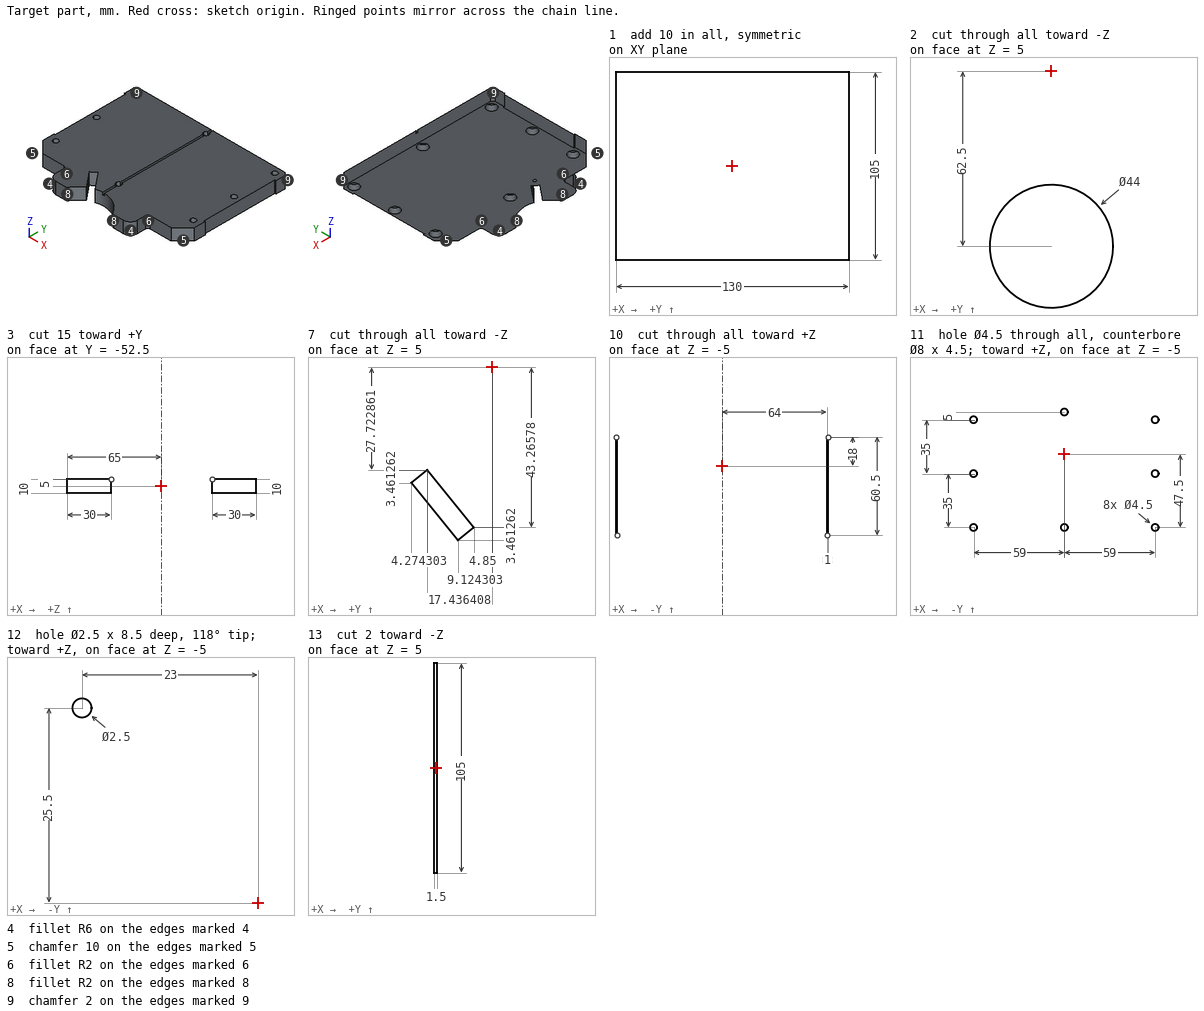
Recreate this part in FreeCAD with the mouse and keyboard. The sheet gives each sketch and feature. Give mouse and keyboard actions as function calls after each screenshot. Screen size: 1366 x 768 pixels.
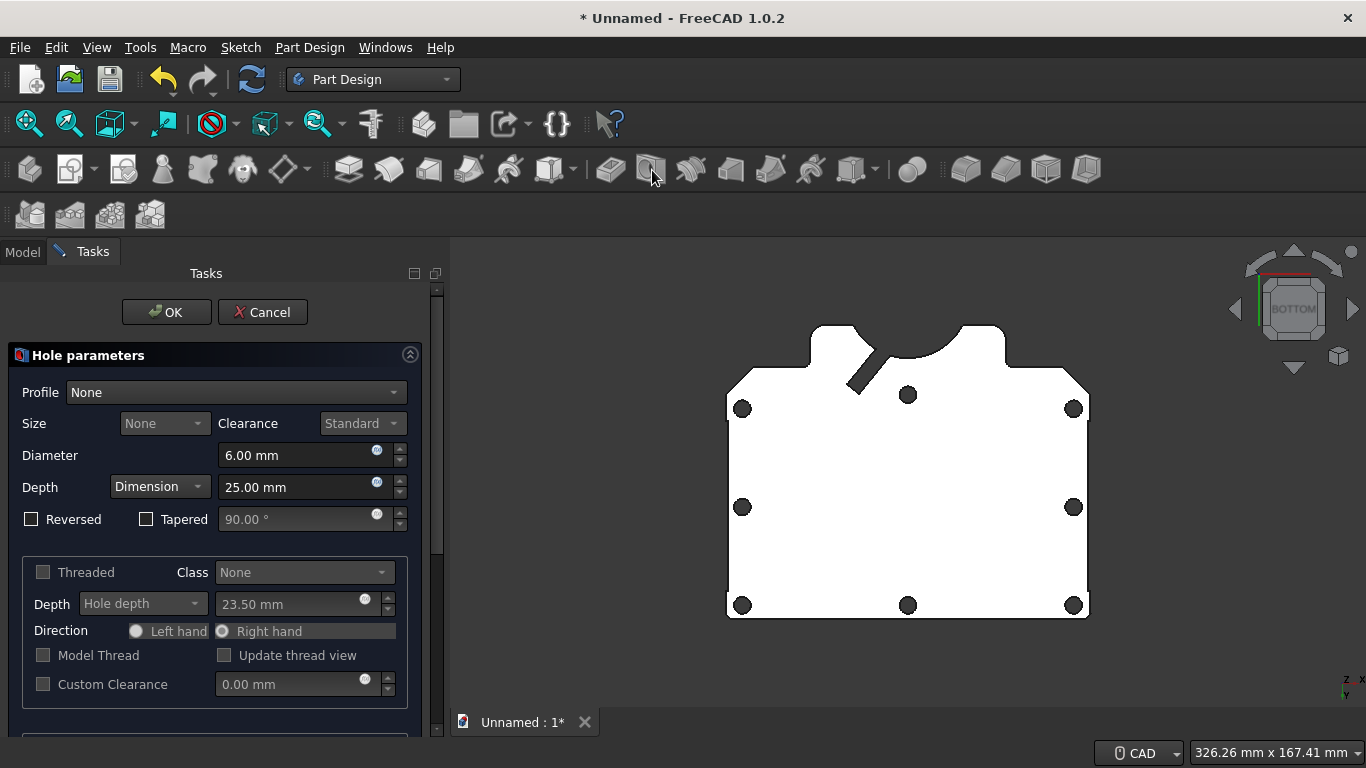
triple_click(305, 455)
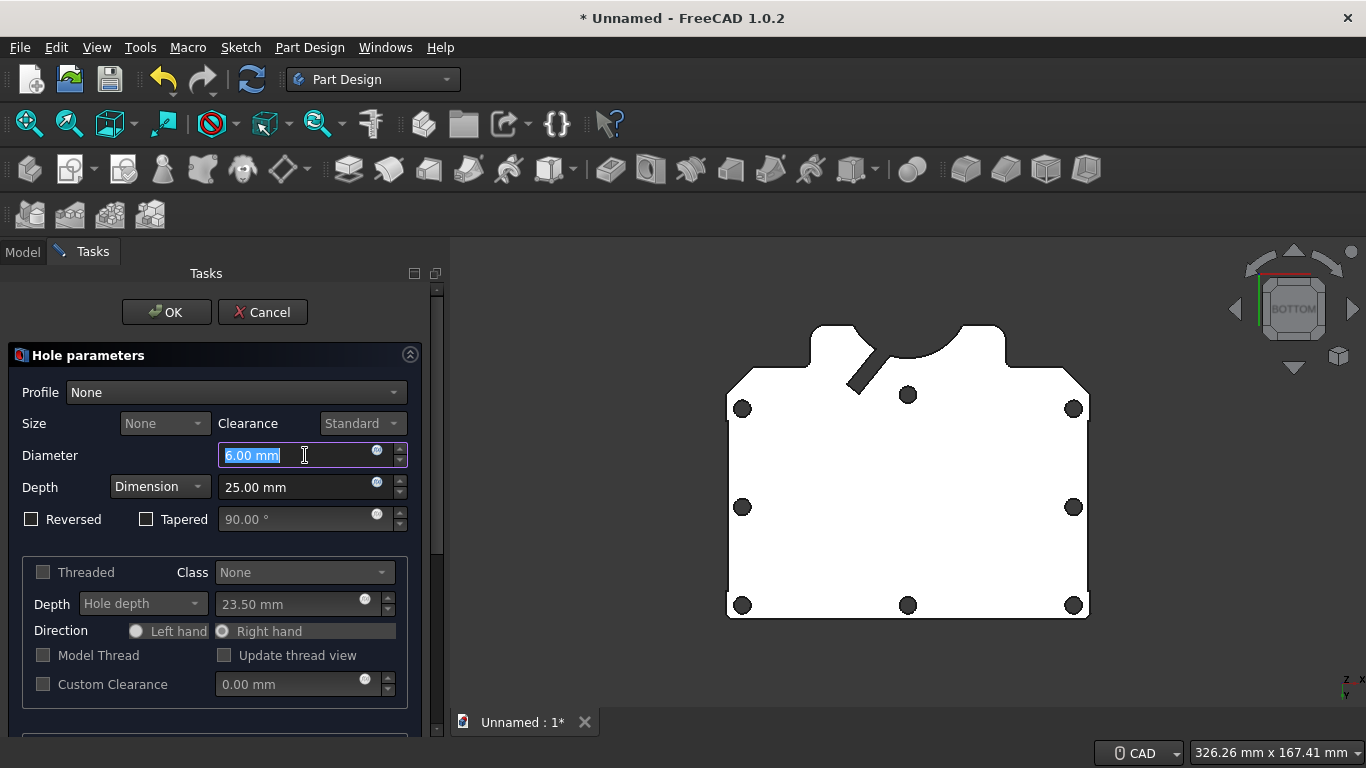
text(4.5)
key(Tab)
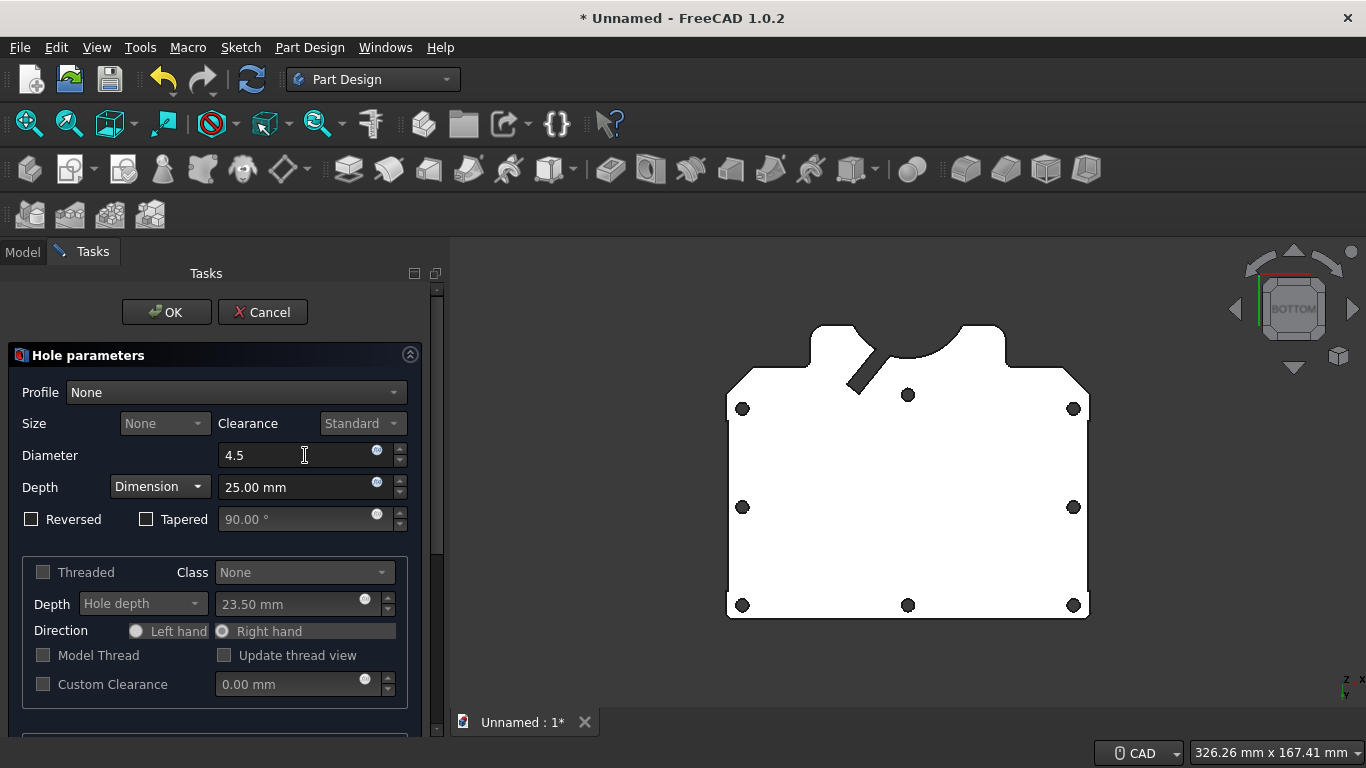
click(161, 486)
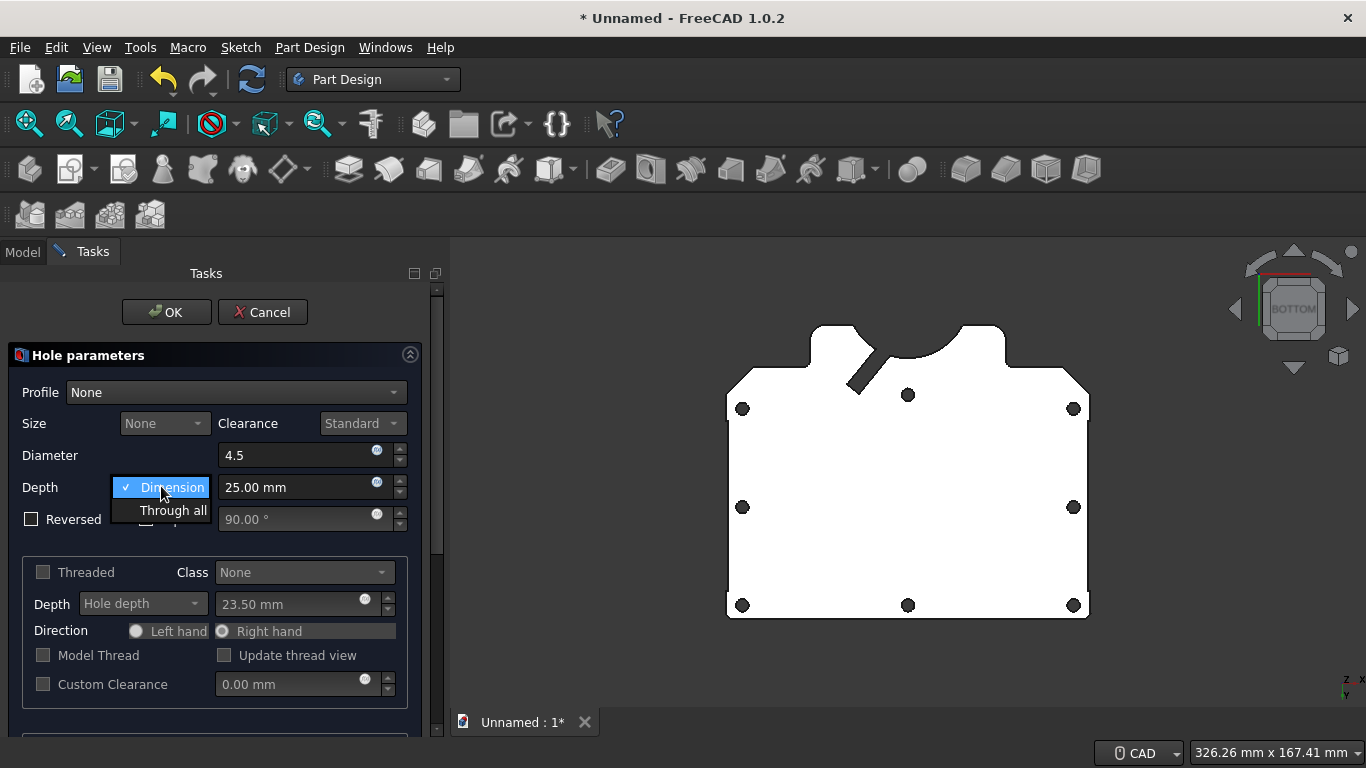
click(160, 510)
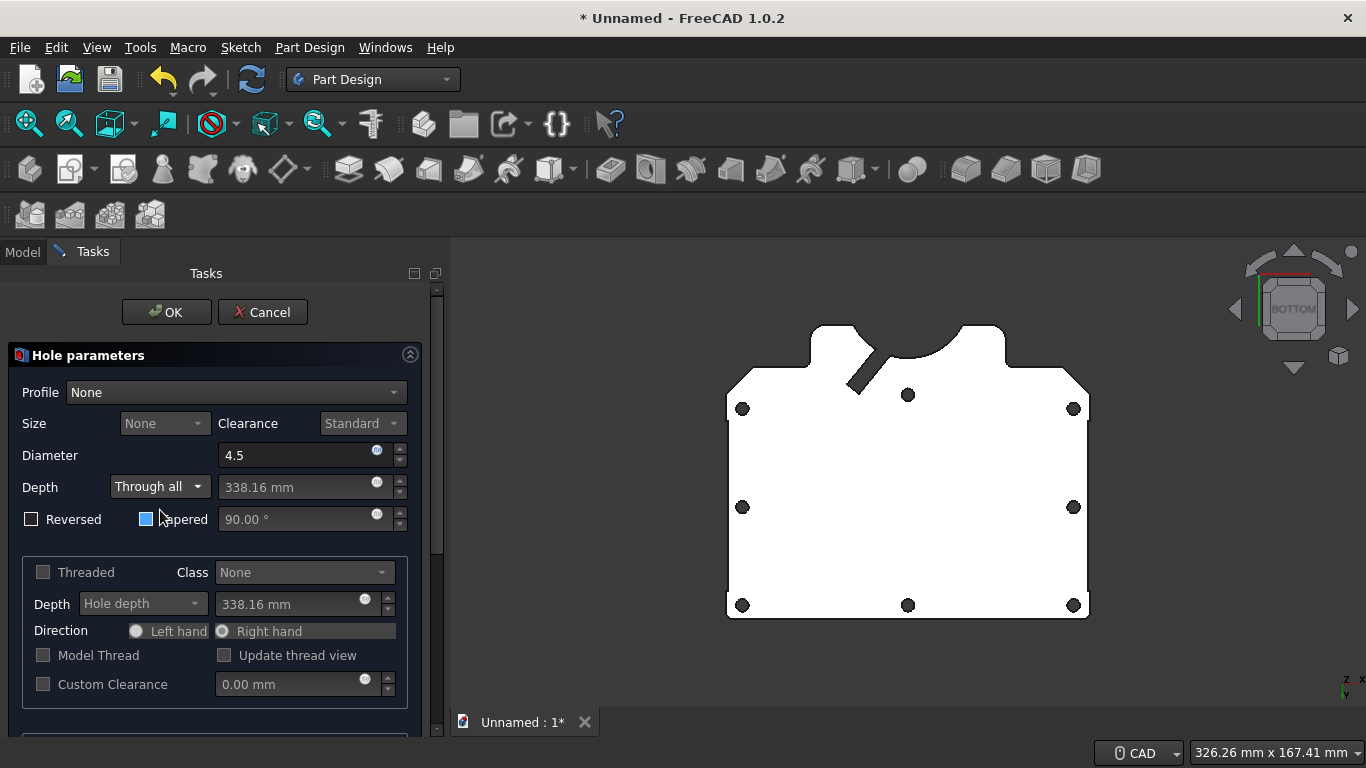
scroll(437, 510, down, 2)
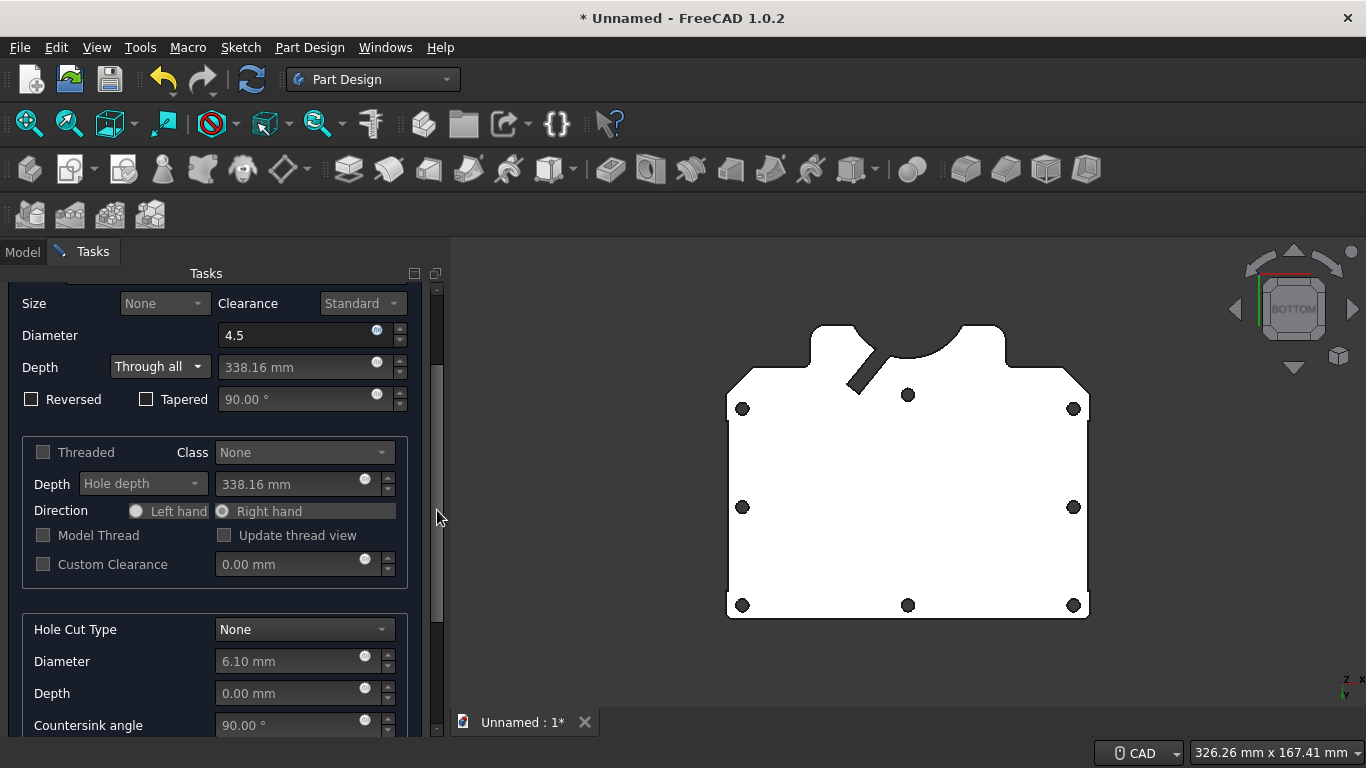
click(306, 630)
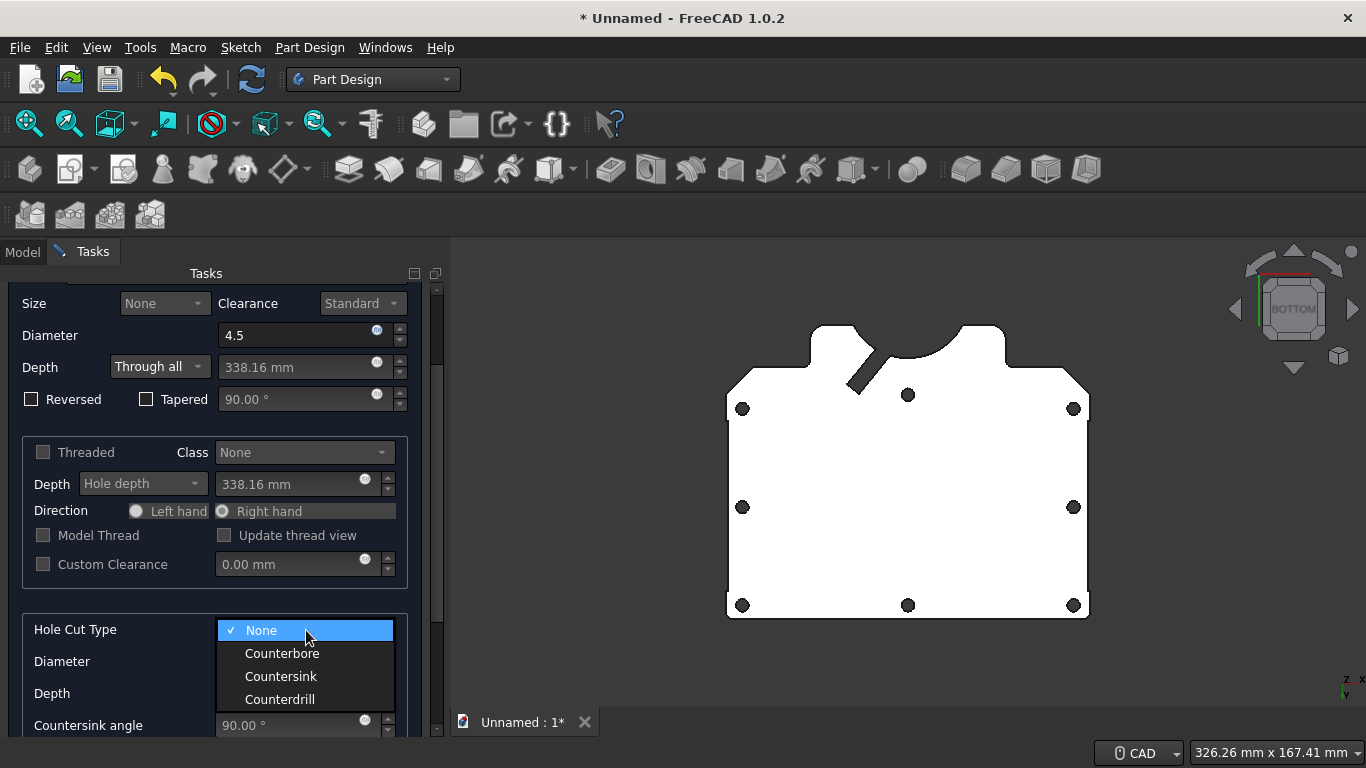
click(304, 654)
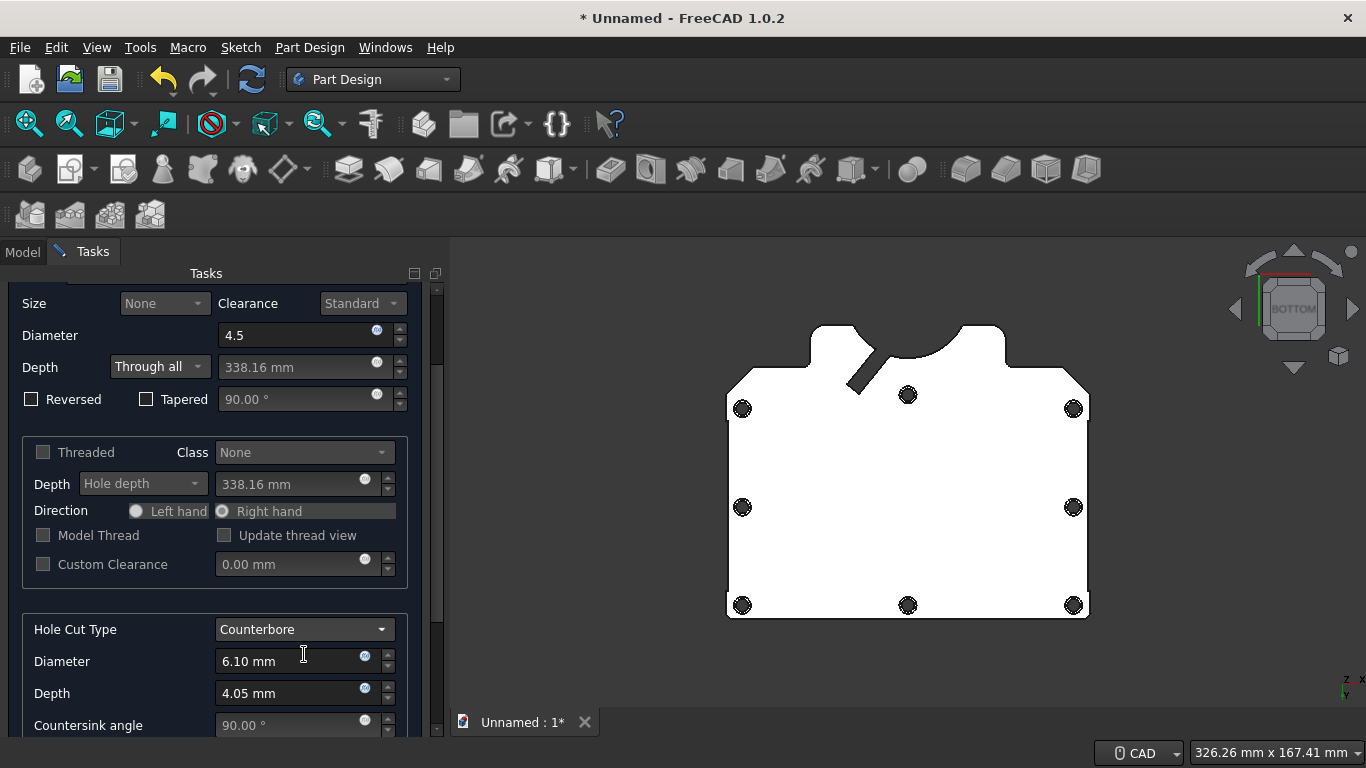
triple_click(298, 661)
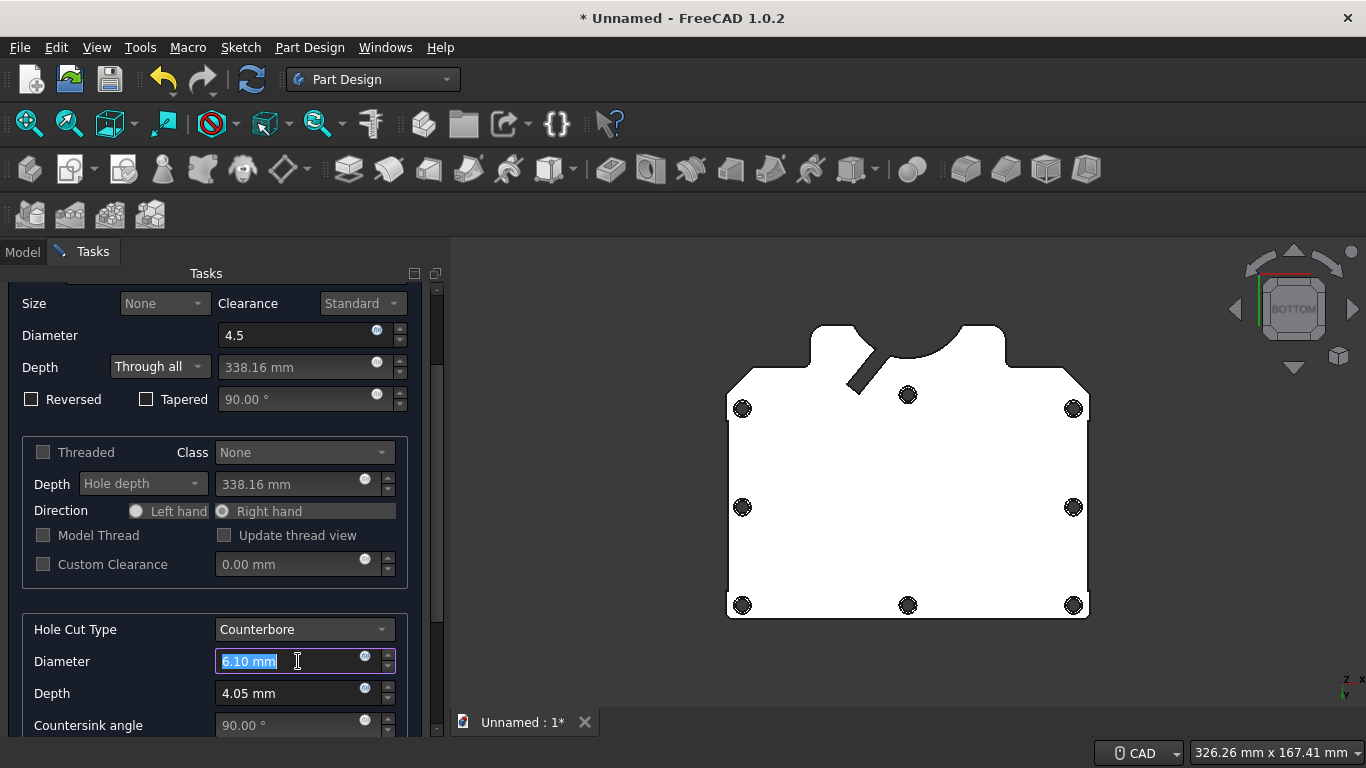
text(8)
key(Tab)